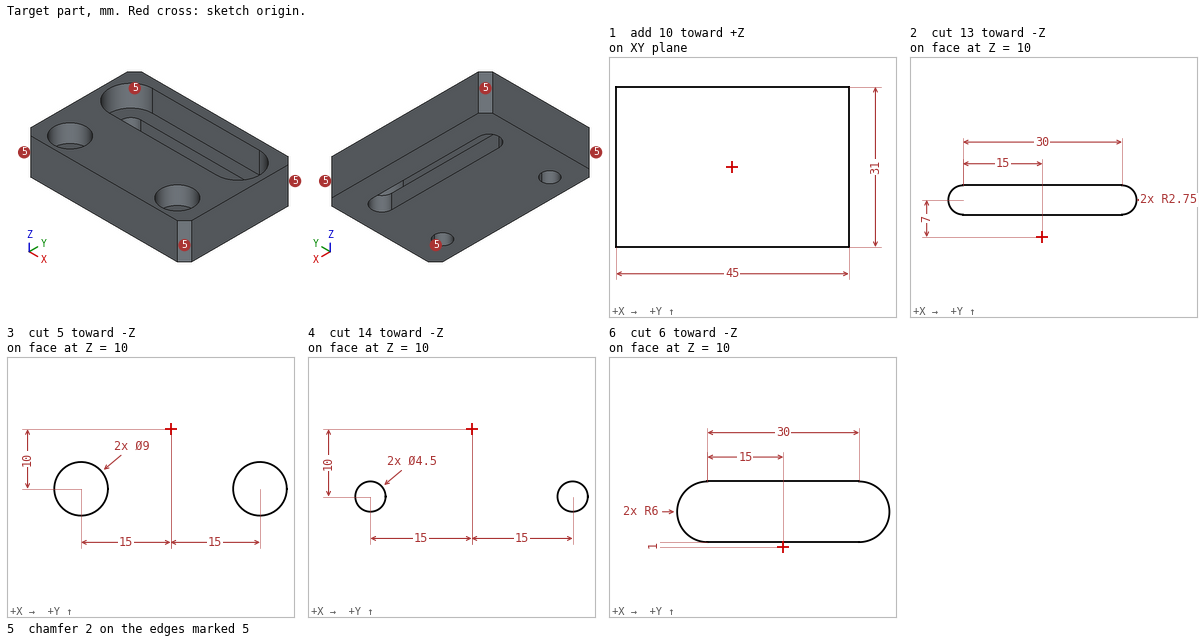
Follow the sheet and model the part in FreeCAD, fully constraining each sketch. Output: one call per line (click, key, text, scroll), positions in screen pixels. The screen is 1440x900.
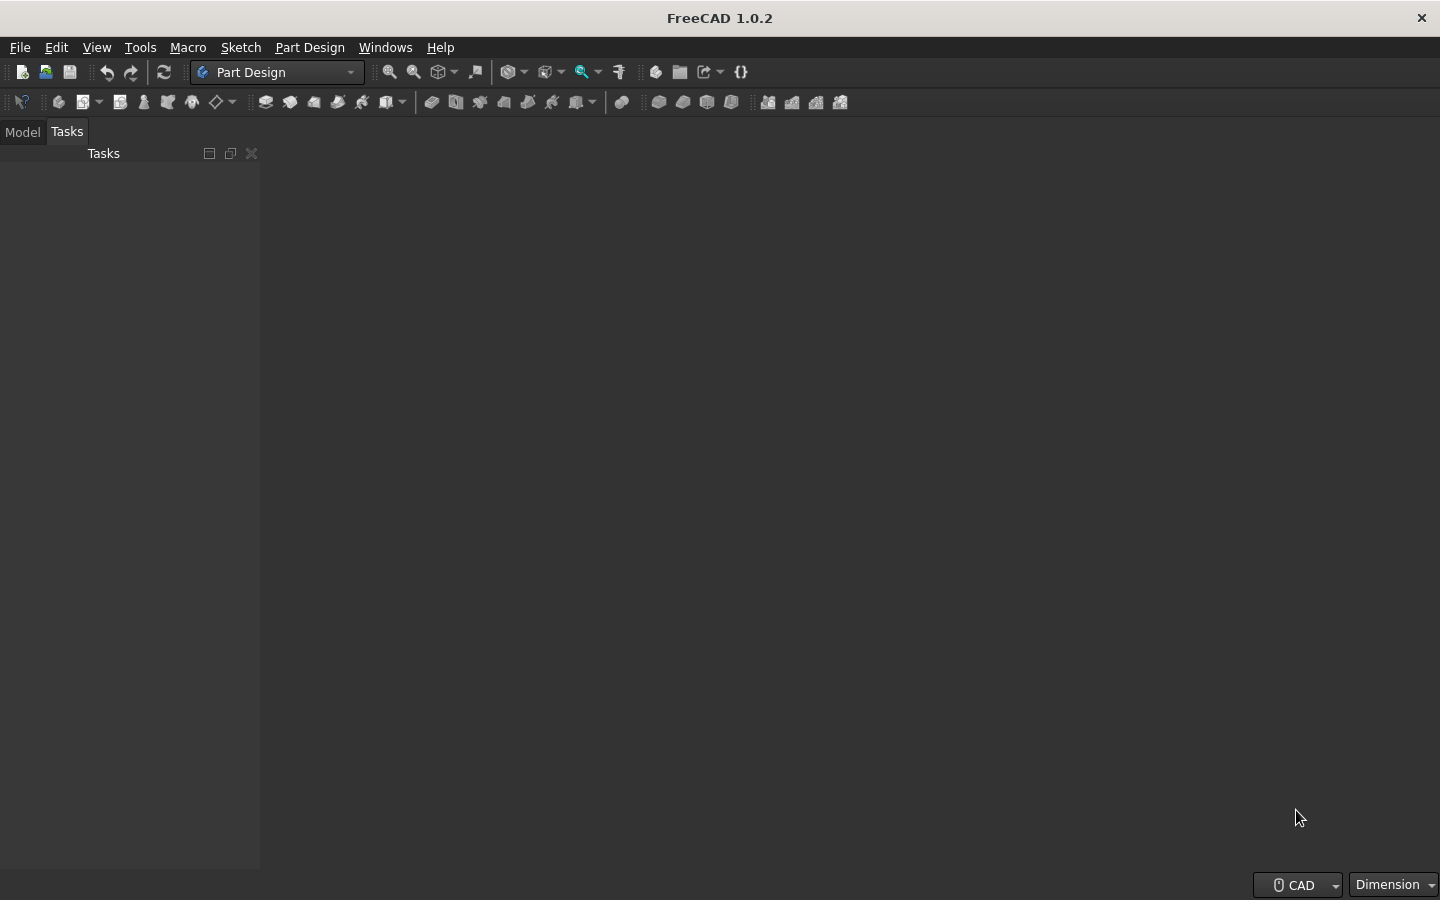
click(288, 102)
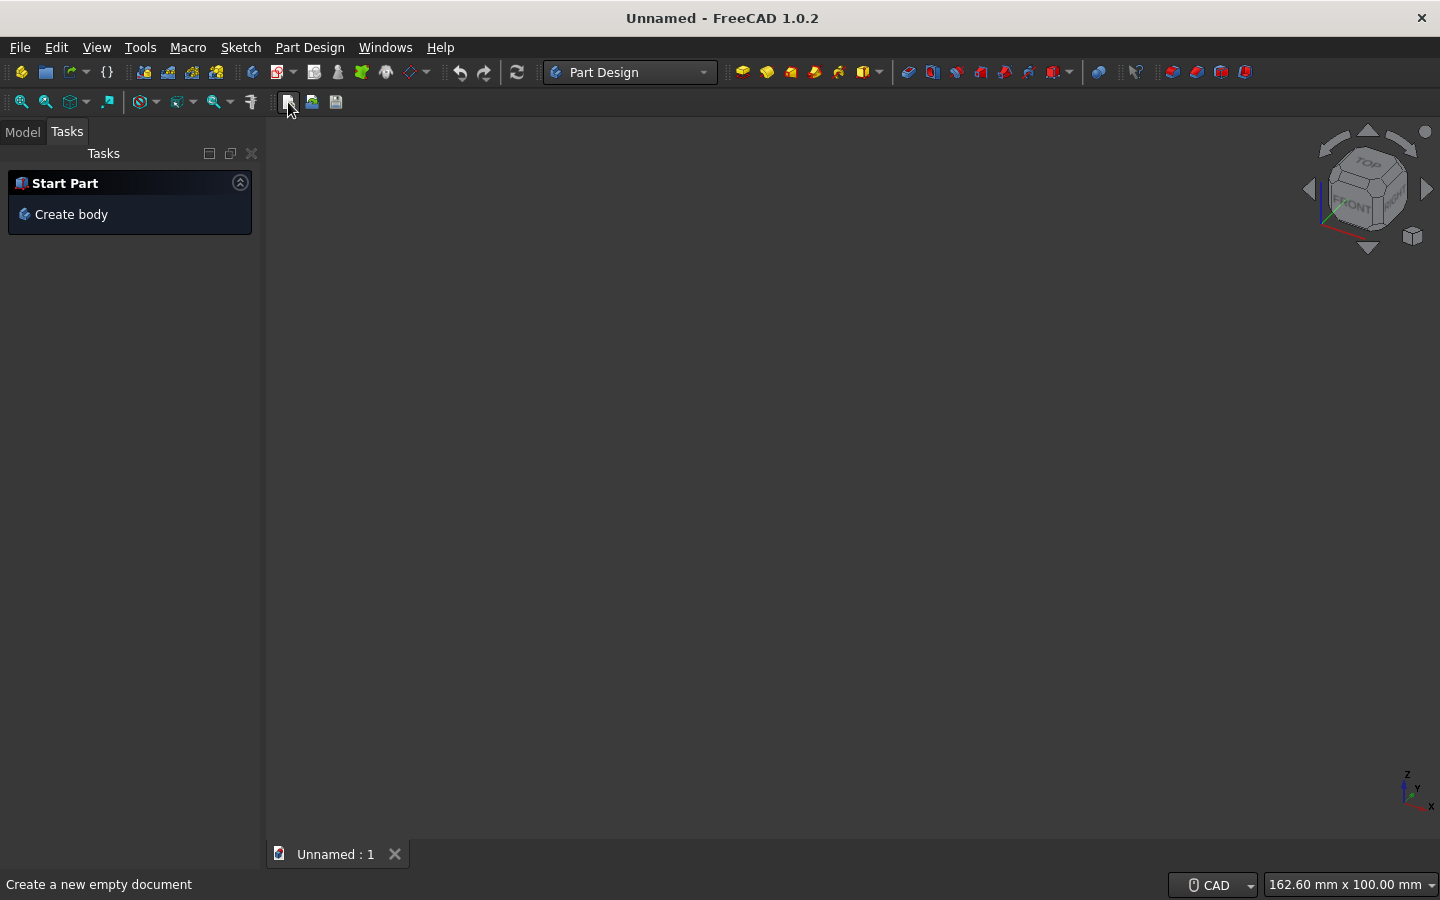
click(278, 72)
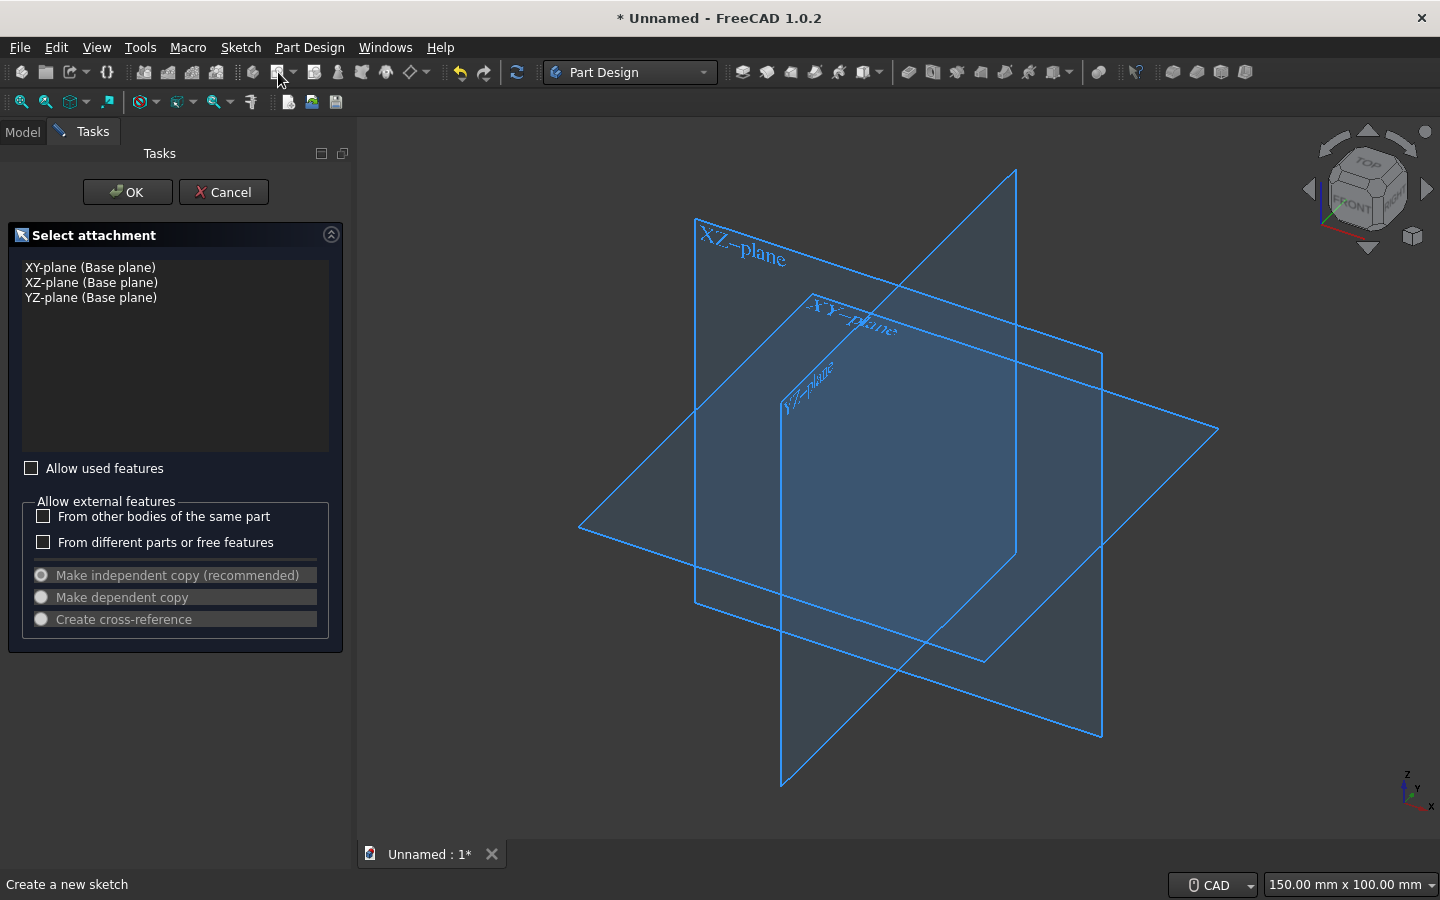
click(82, 268)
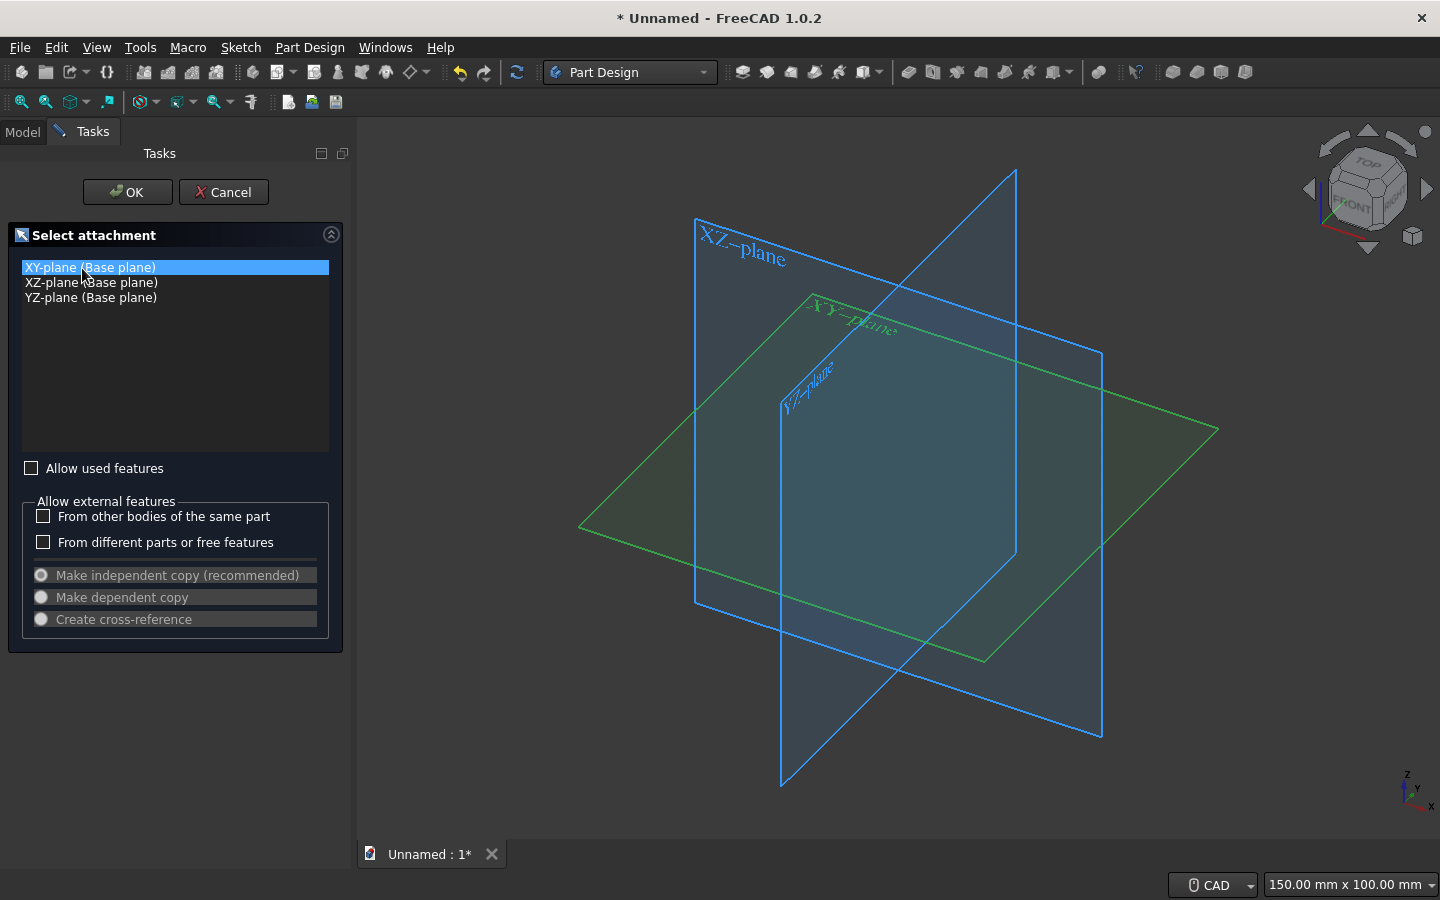
click(128, 192)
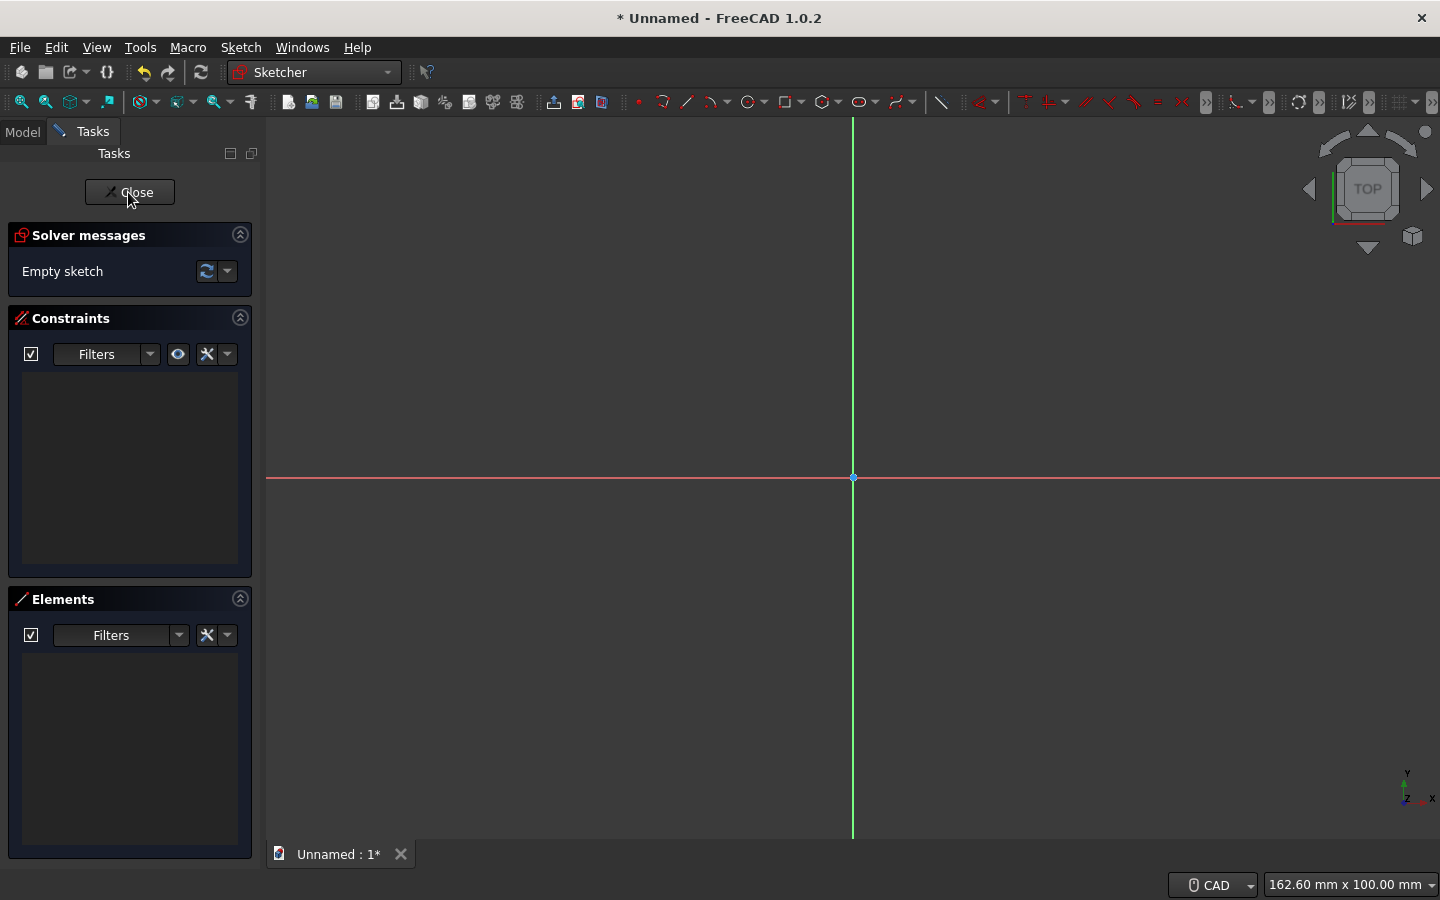
scroll(909, 478, up, 4)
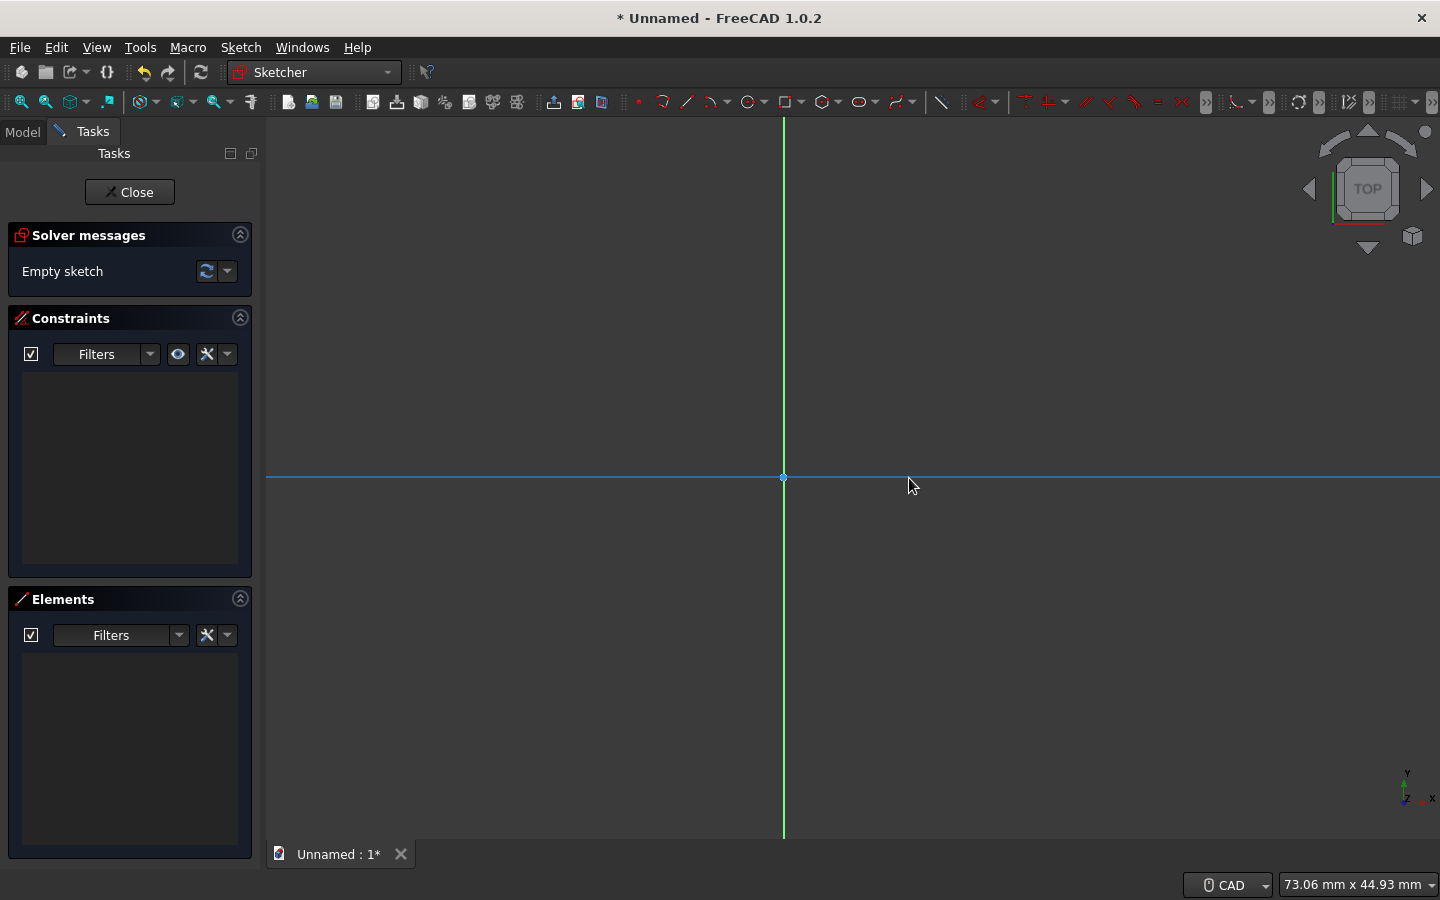
click(804, 102)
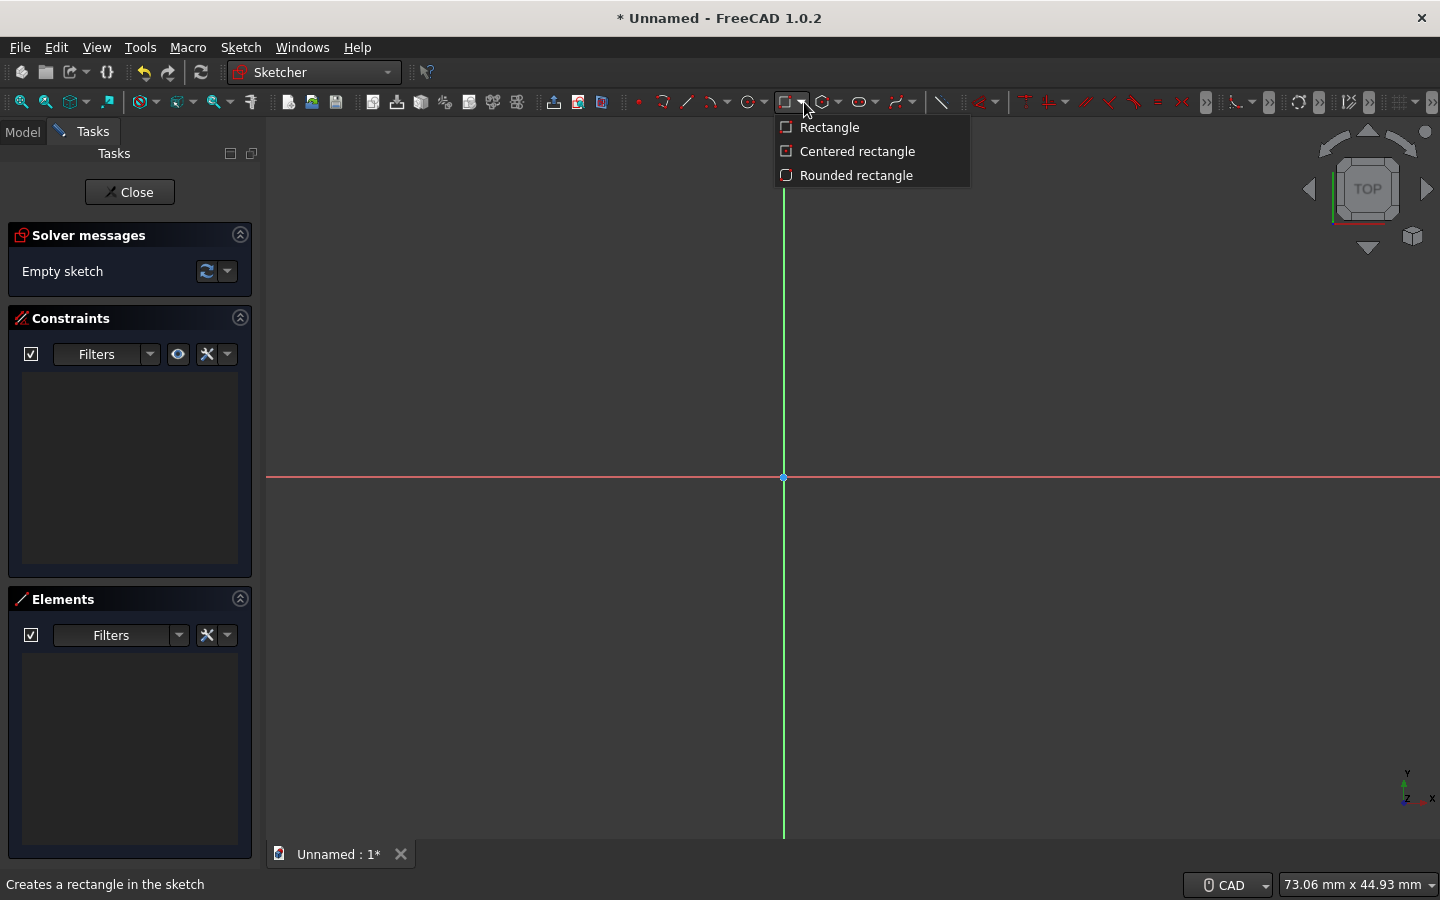
click(872, 151)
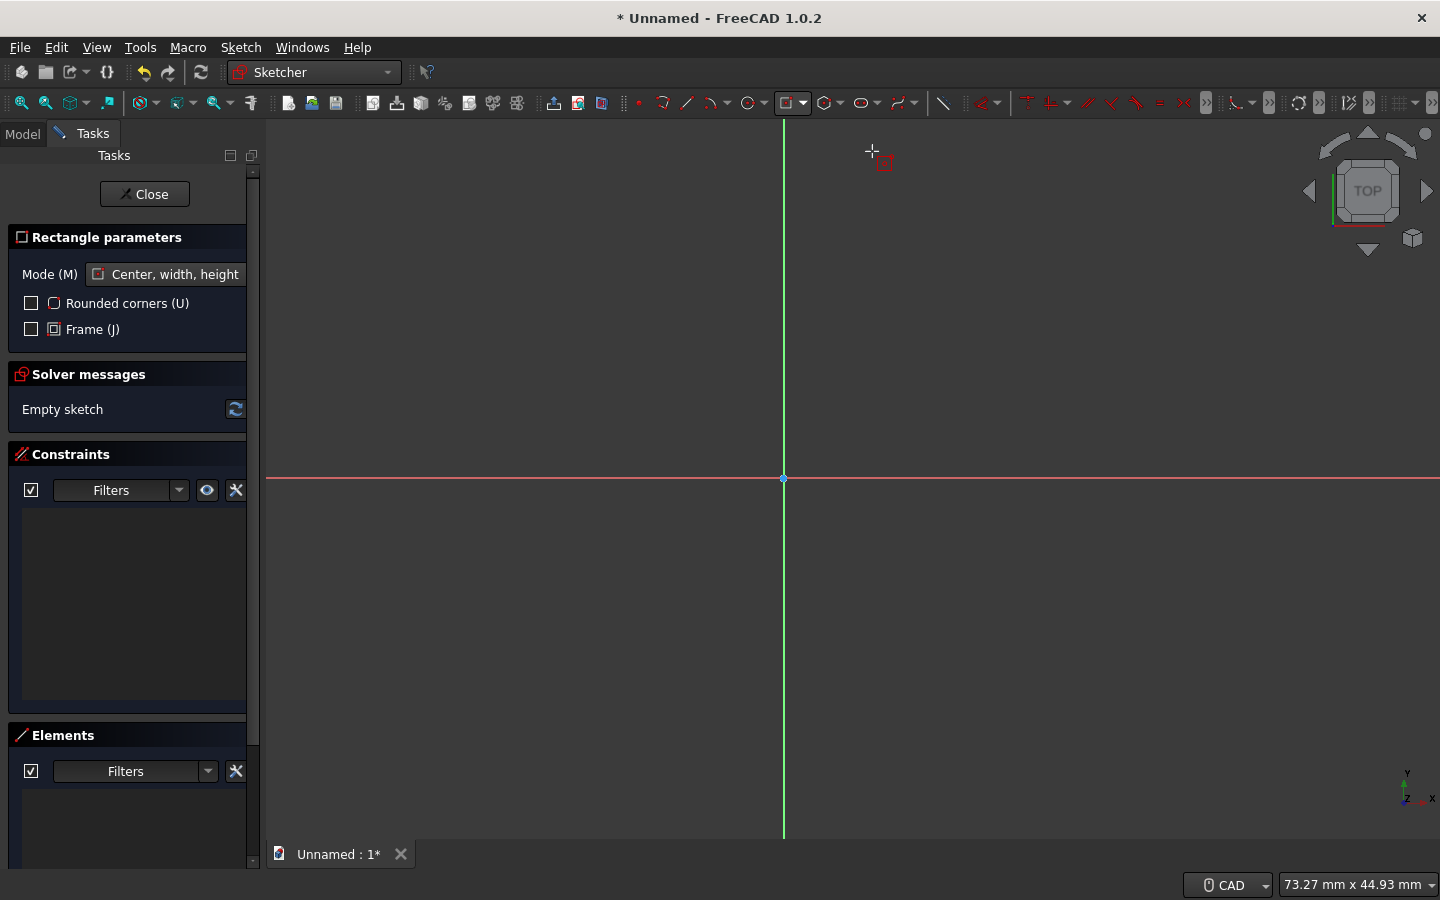
click(784, 478)
click(1144, 230)
key(Escape)